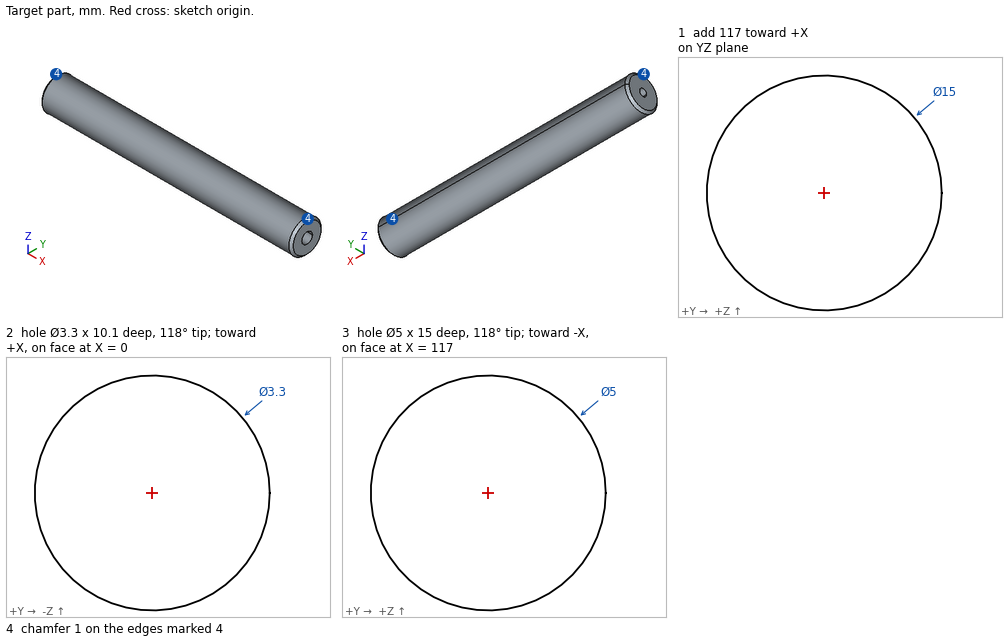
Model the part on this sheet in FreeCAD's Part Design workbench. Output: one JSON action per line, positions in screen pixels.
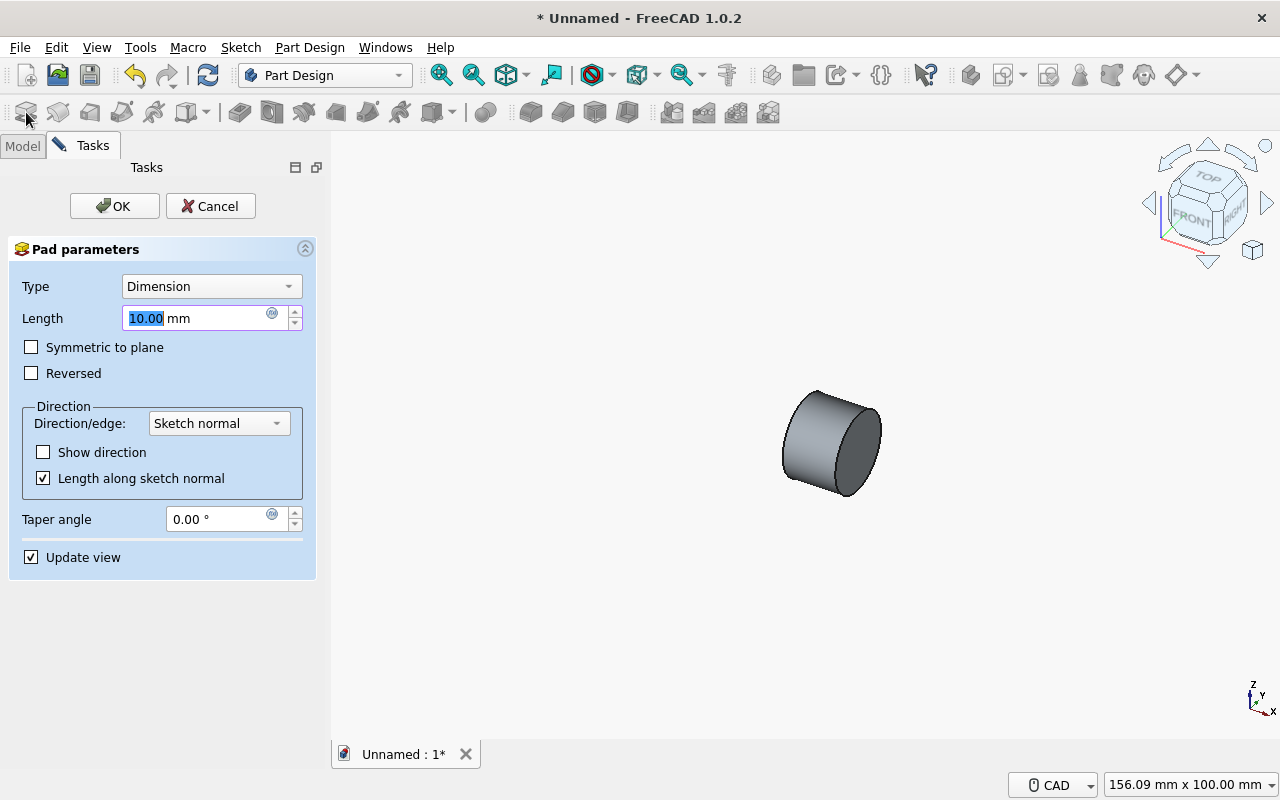
{"action": "type", "text": "117"}
{"action": "key", "text": "Tab"}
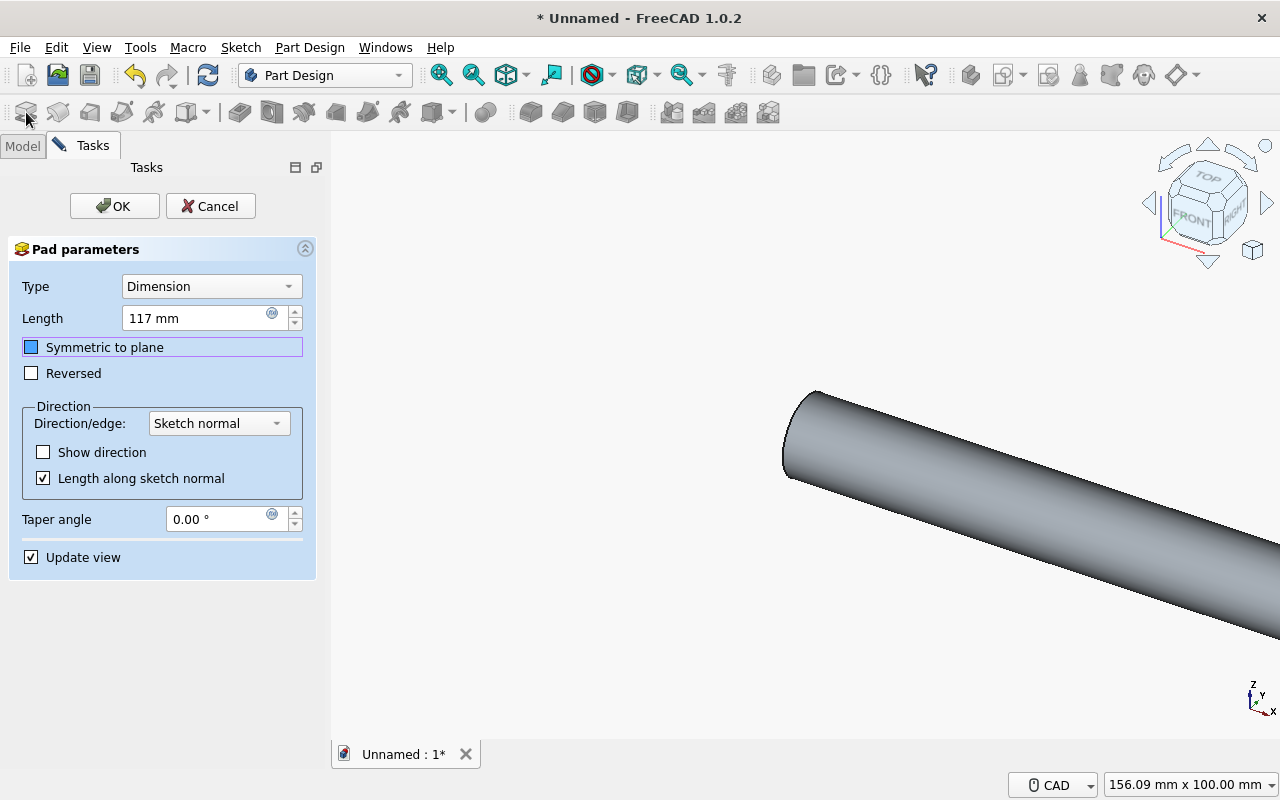
{"action": "left_click", "coordinate": [115, 206]}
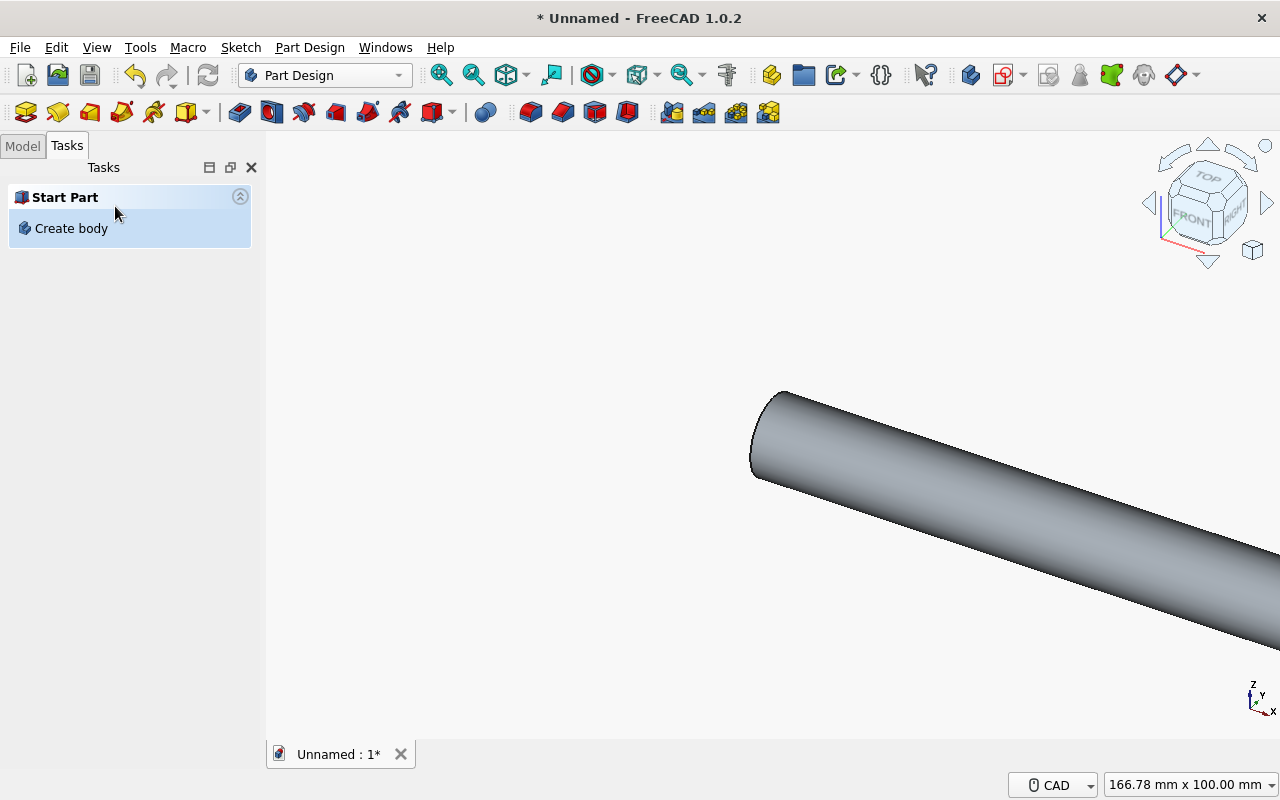
{"action": "left_click", "coordinate": [442, 76]}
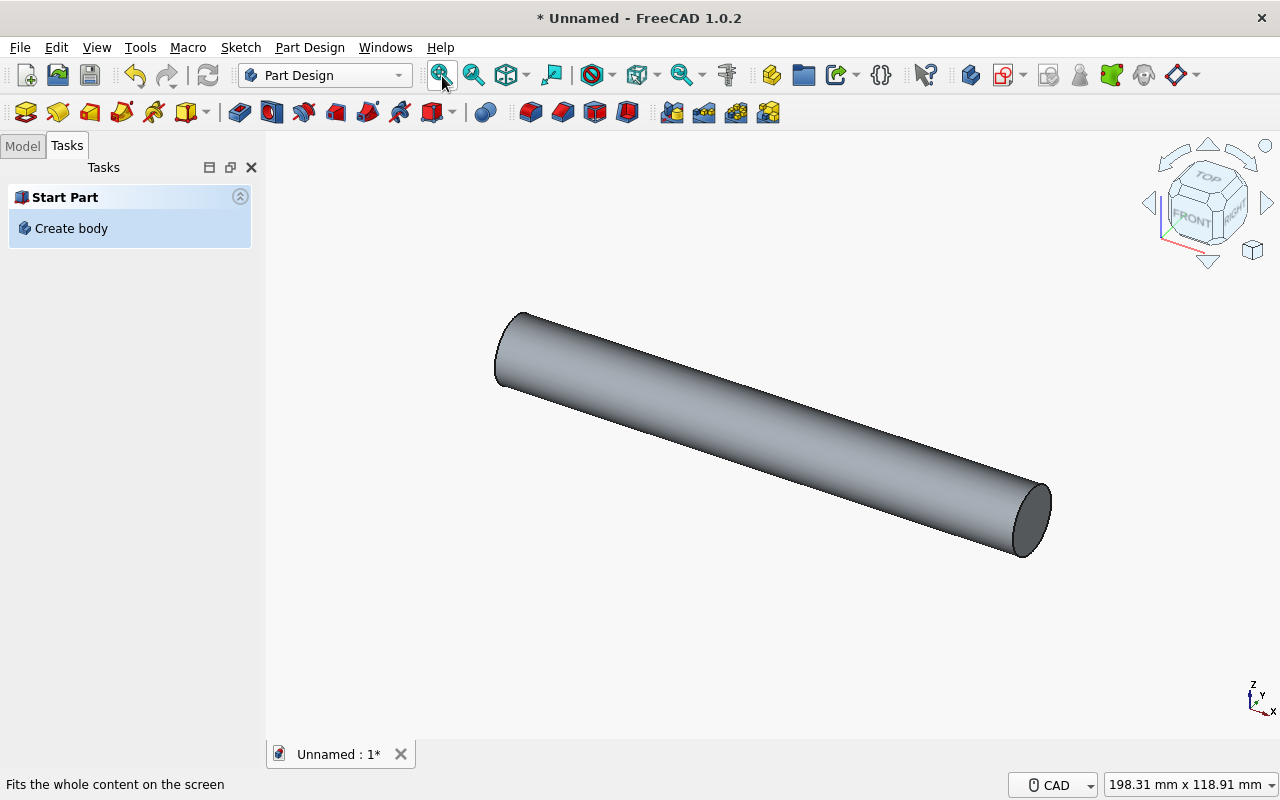
{"action": "key", "text": "6"}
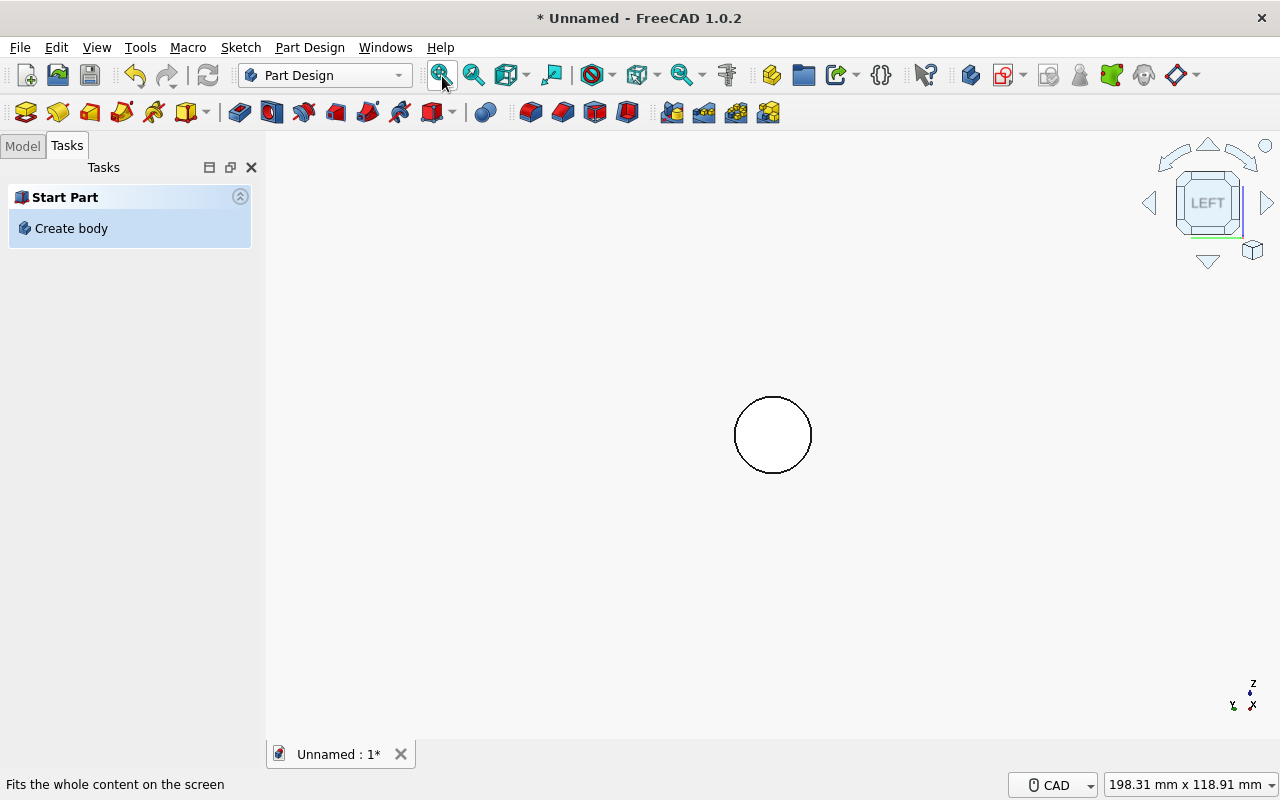
{"action": "left_click", "coordinate": [442, 76]}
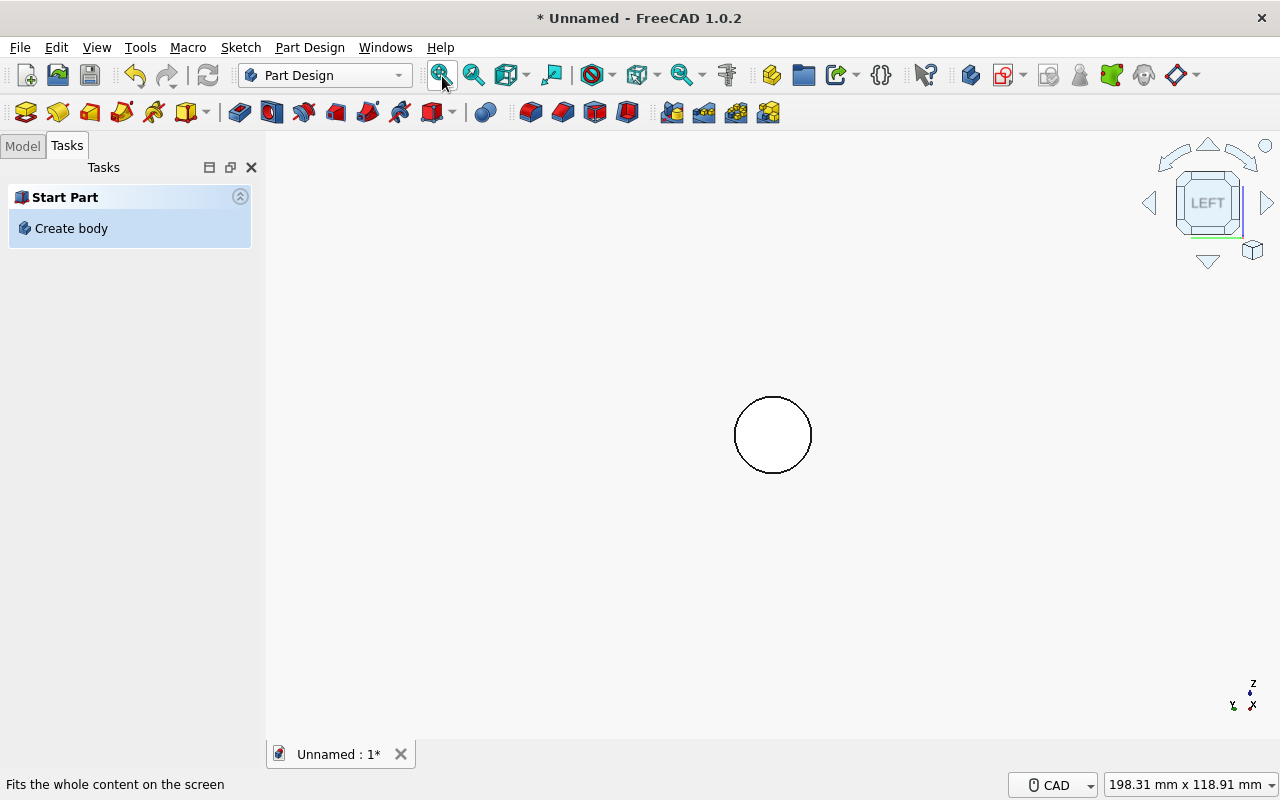
{"action": "left_click", "coordinate": [773, 434]}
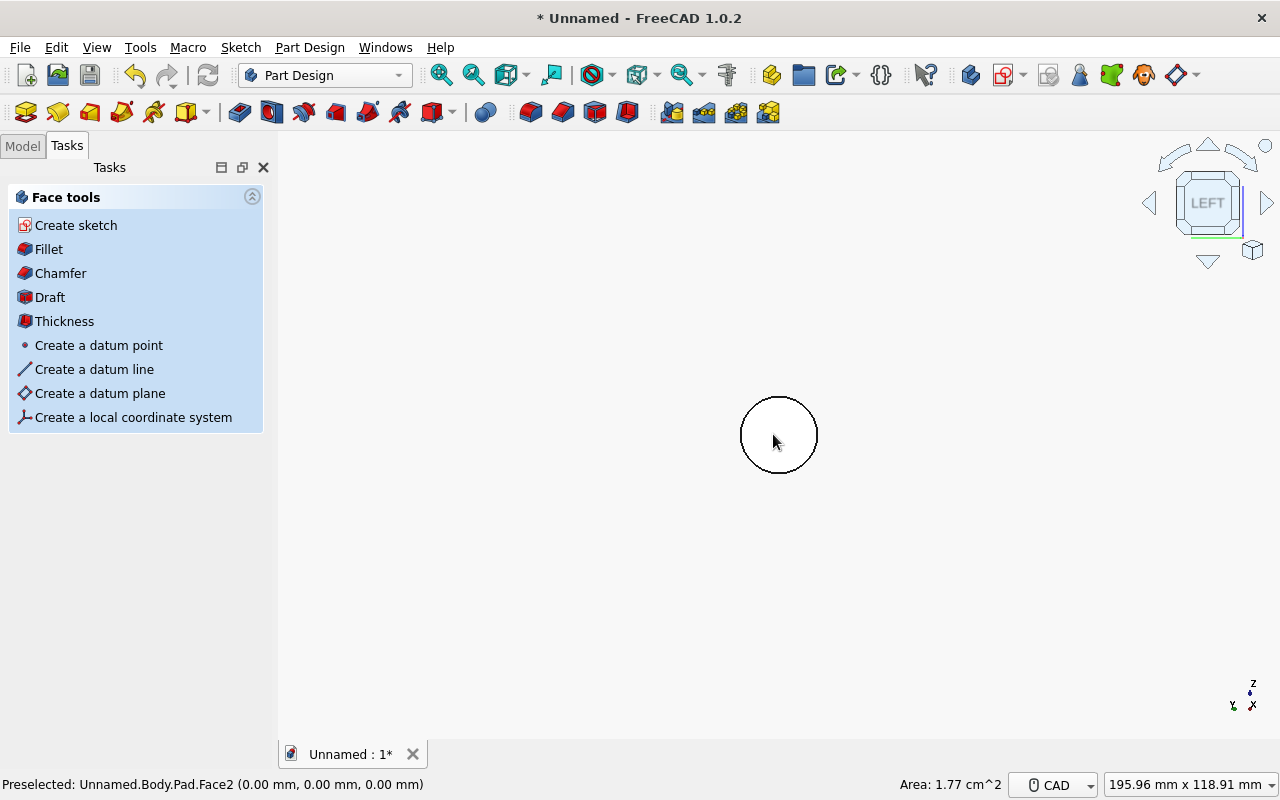
{"action": "left_click", "coordinate": [1004, 76]}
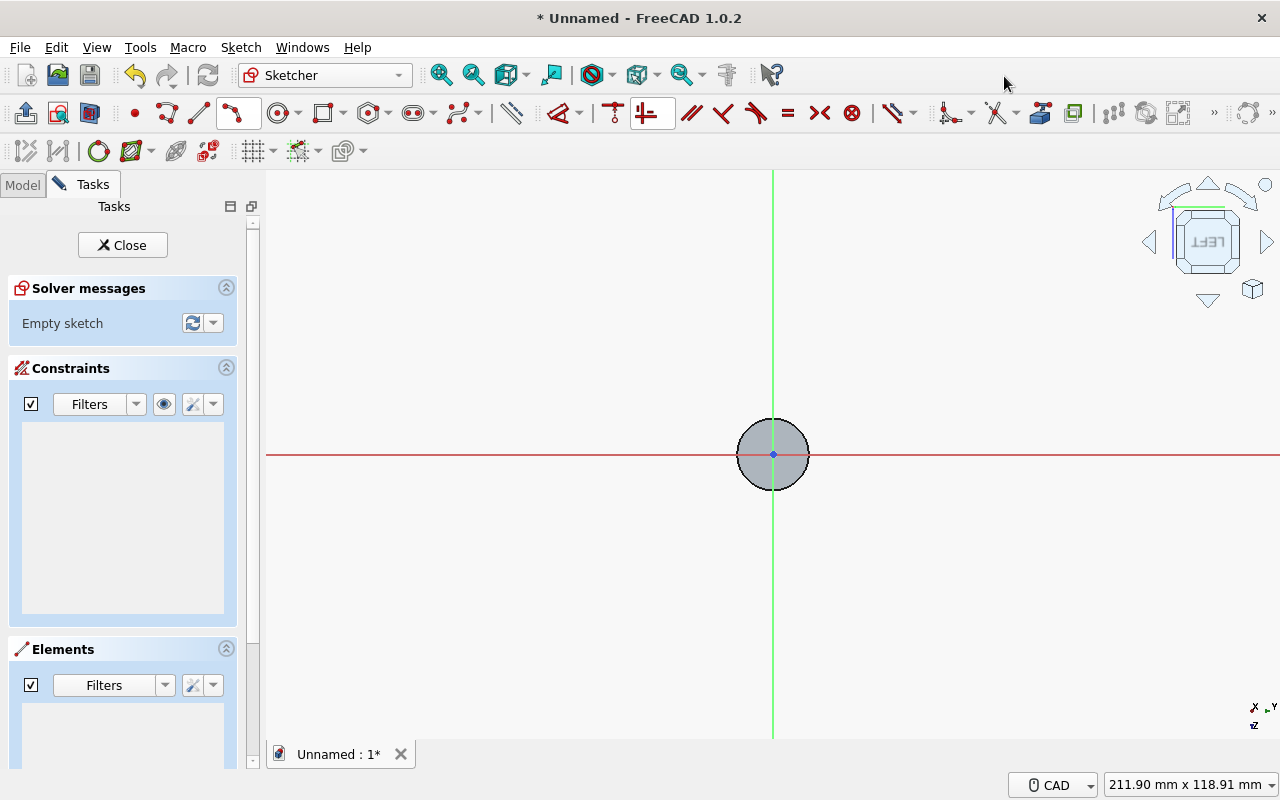
{"action": "scroll", "coordinate": [777, 455], "scroll_direction": "up", "scroll_amount": 15}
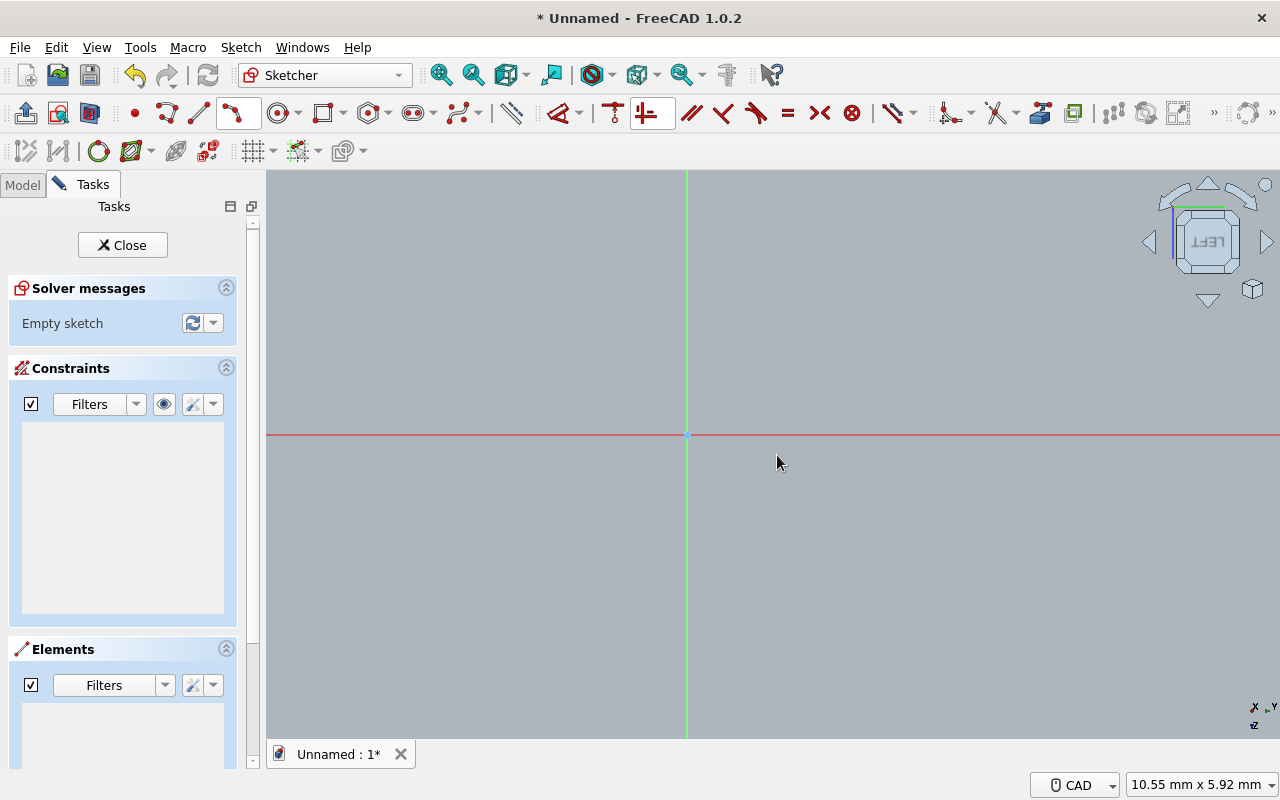
{"action": "left_click", "coordinate": [278, 114]}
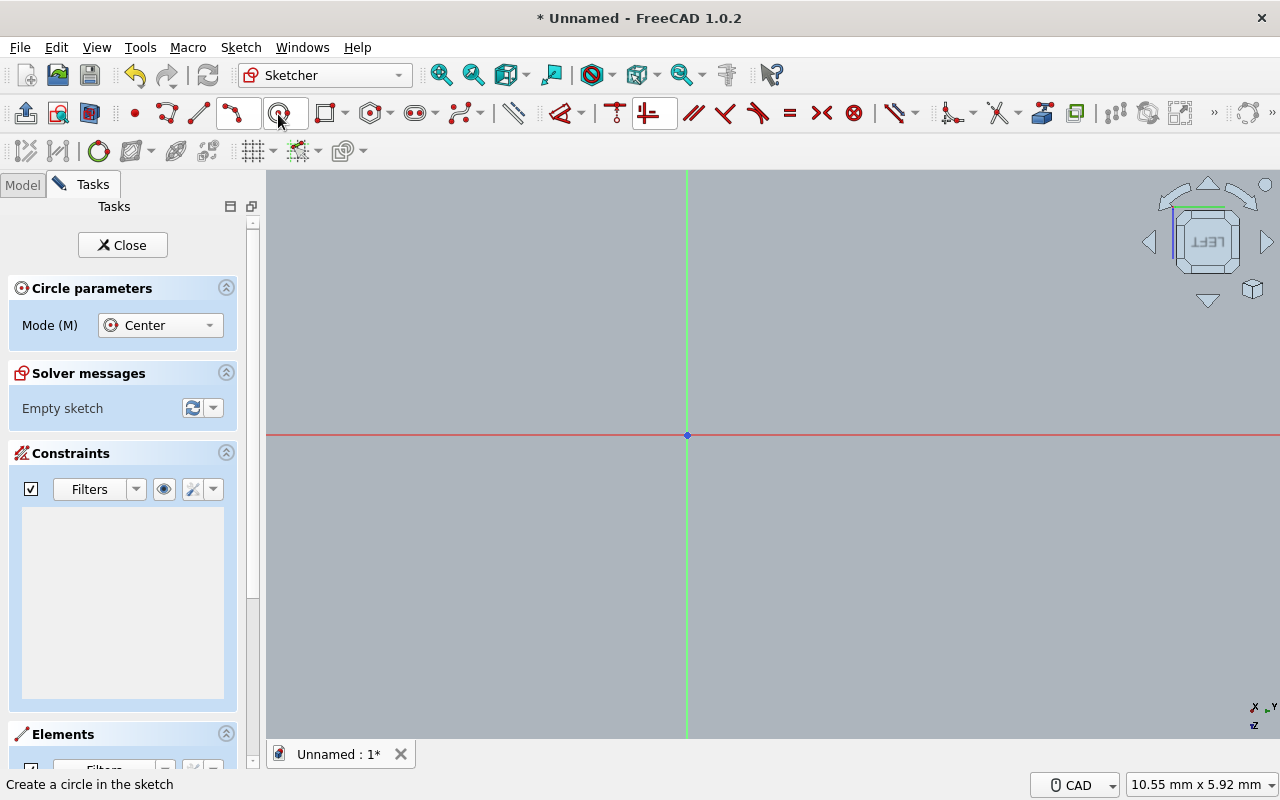
{"action": "left_click", "coordinate": [687, 435]}
{"action": "mouse_move", "coordinate": [799, 323]}